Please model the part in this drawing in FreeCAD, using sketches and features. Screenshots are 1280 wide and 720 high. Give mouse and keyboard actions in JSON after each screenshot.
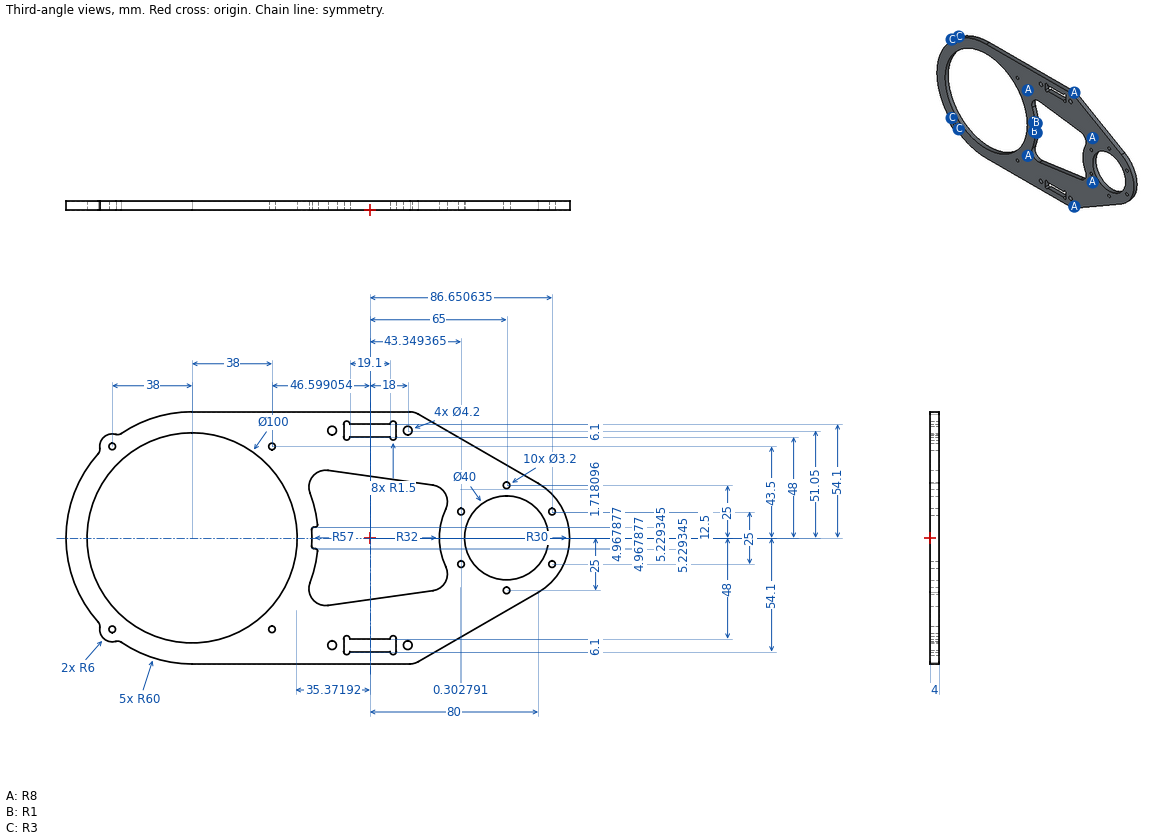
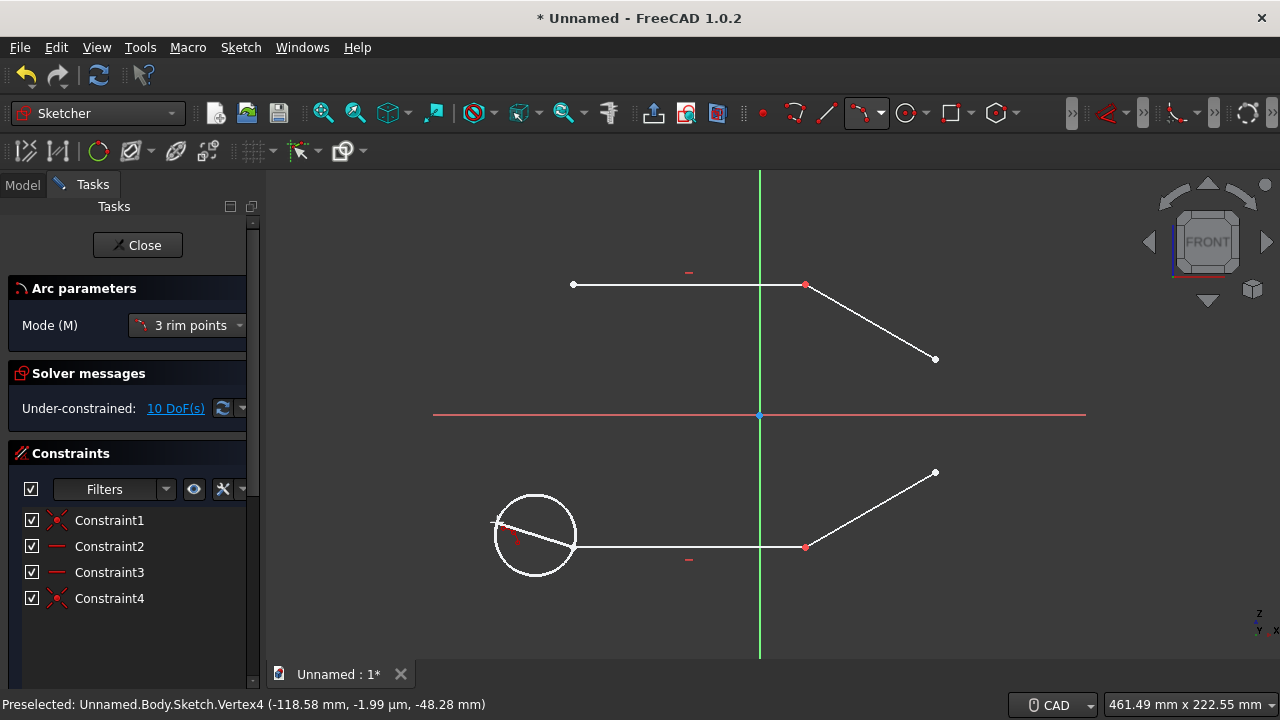
{"action": "scroll", "coordinate": [533, 541], "scroll_direction": "up", "scroll_amount": 5}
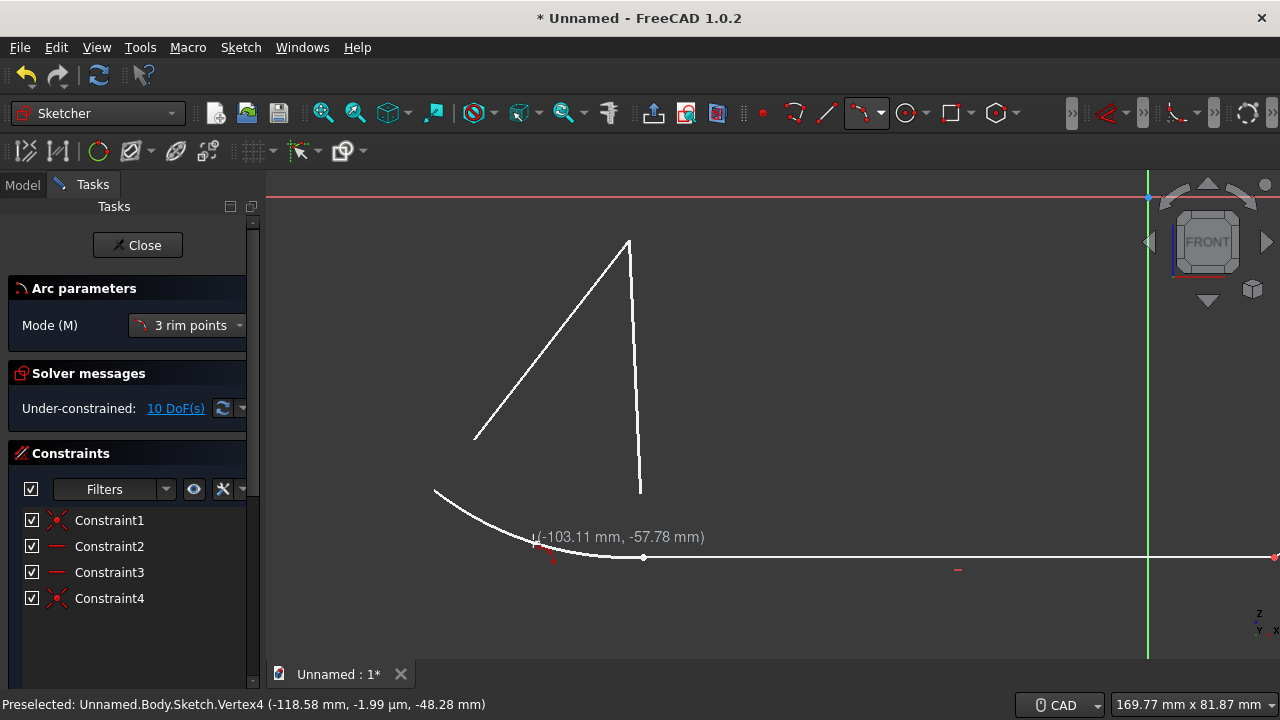
{"action": "left_click", "coordinate": [533, 538]}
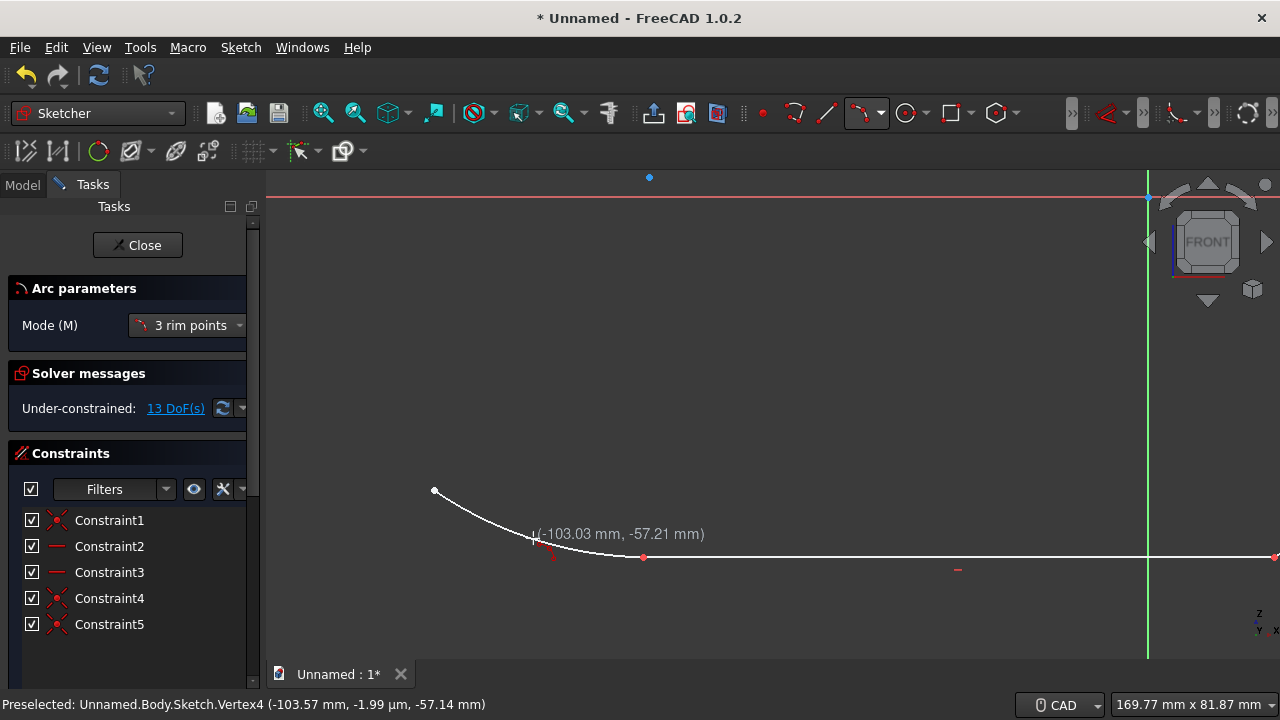
{"action": "left_click", "coordinate": [435, 491]}
{"action": "left_click", "coordinate": [383, 444]}
{"action": "left_click", "coordinate": [393, 484]}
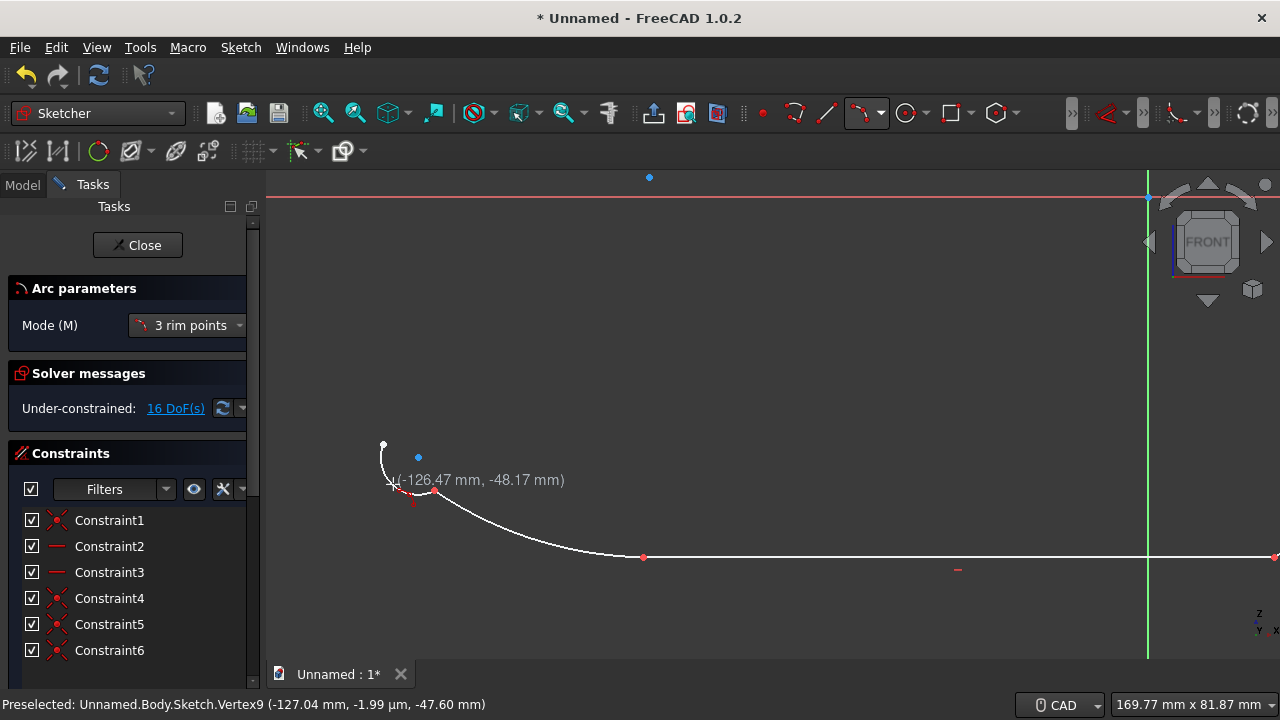
{"action": "left_click", "coordinate": [383, 445]}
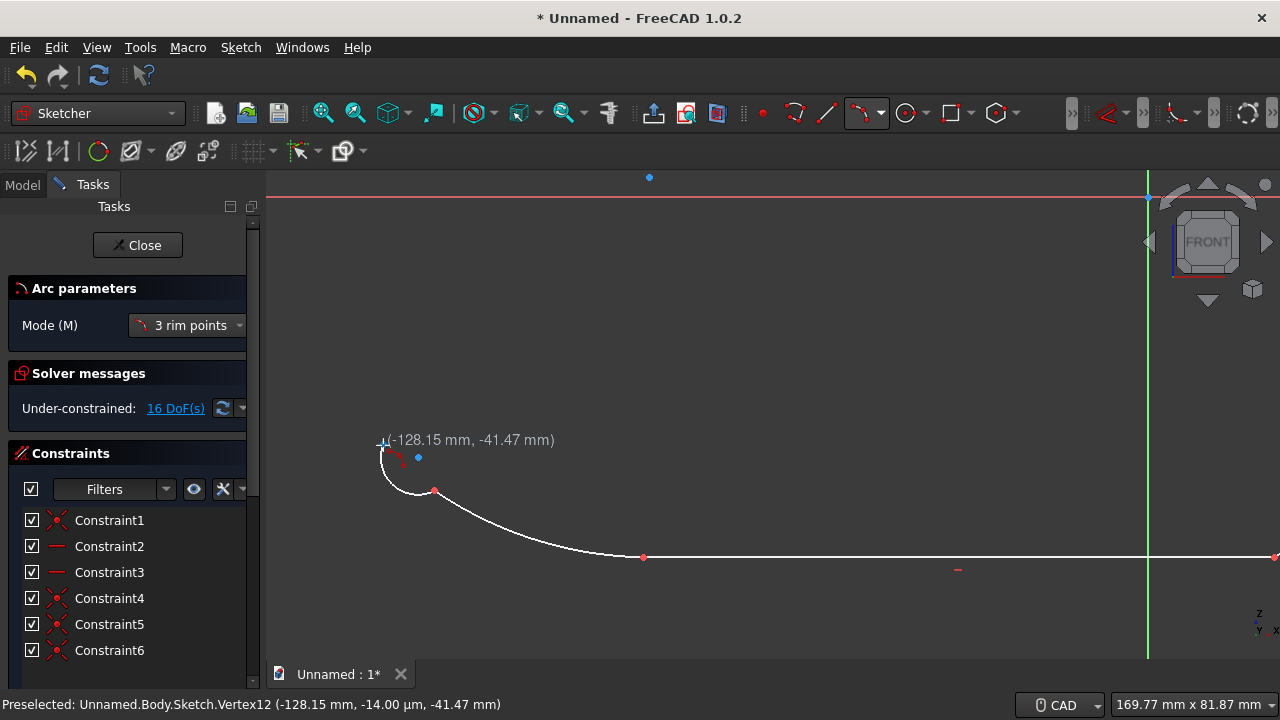
{"action": "scroll", "coordinate": [532, 541], "scroll_direction": "down", "scroll_amount": 5}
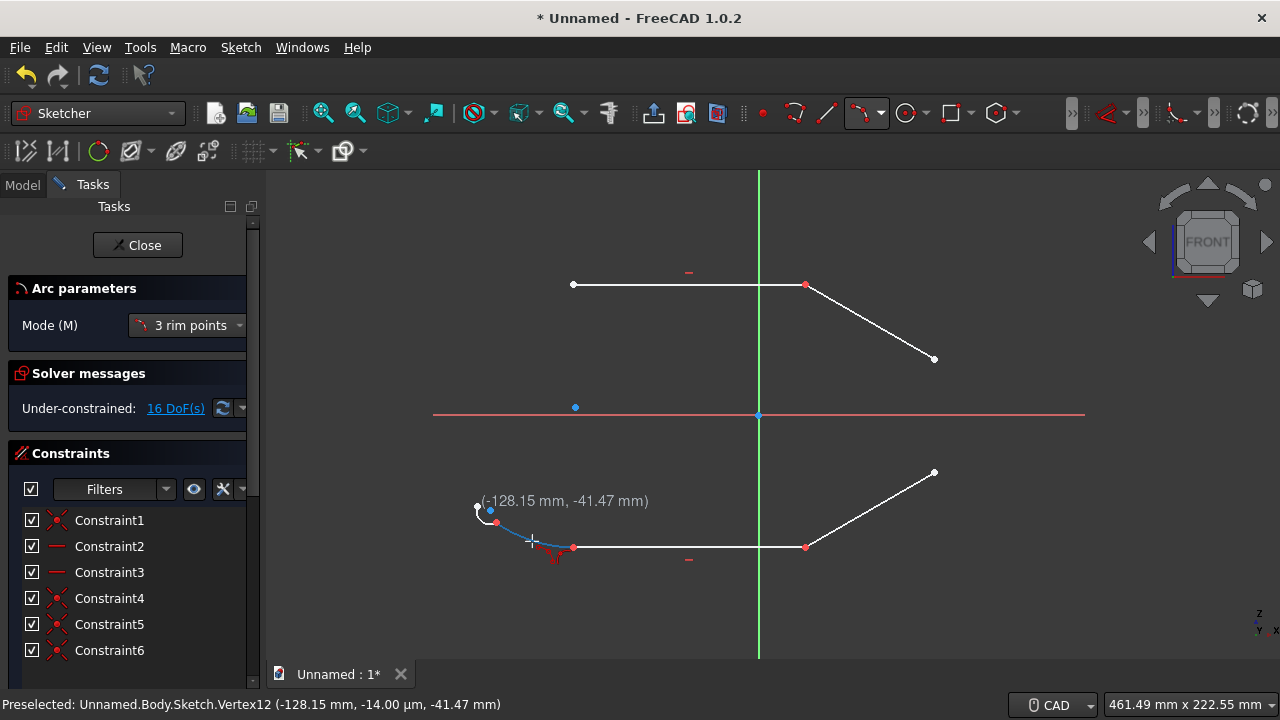
{"action": "left_click", "coordinate": [477, 324]}
{"action": "left_click", "coordinate": [443, 395]}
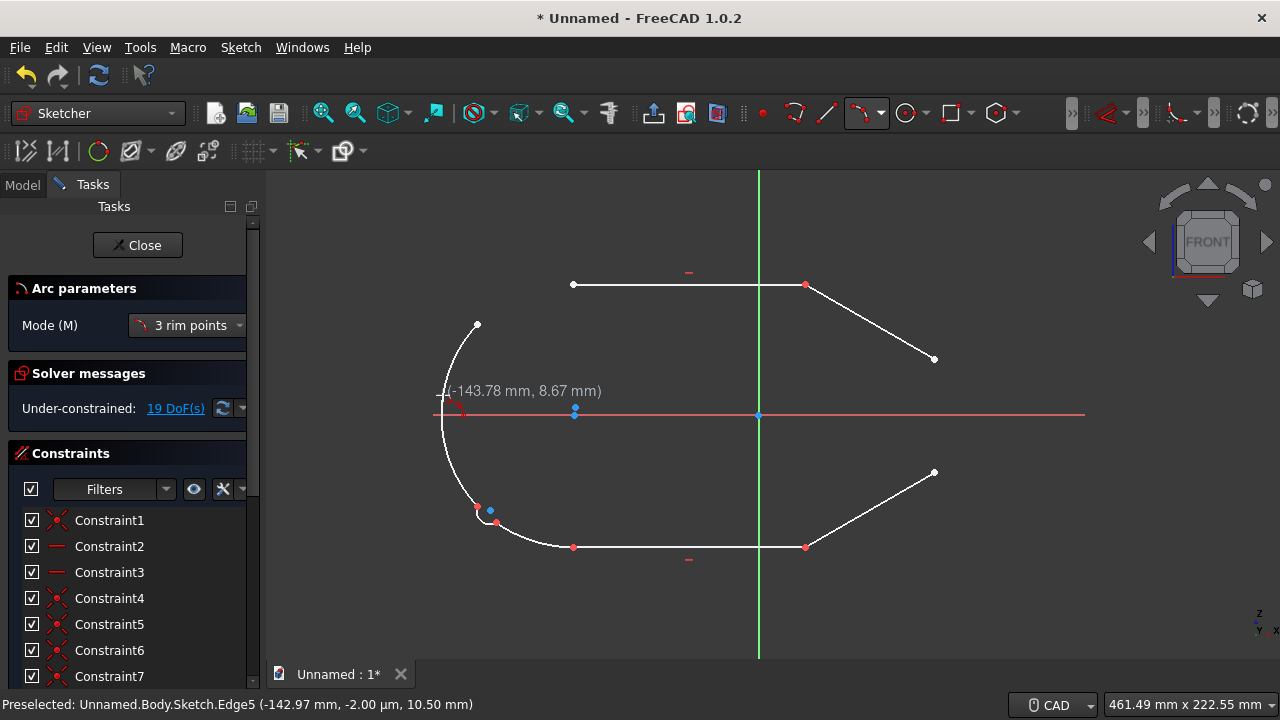
{"action": "left_click", "coordinate": [477, 325]}
{"action": "left_click", "coordinate": [496, 308]}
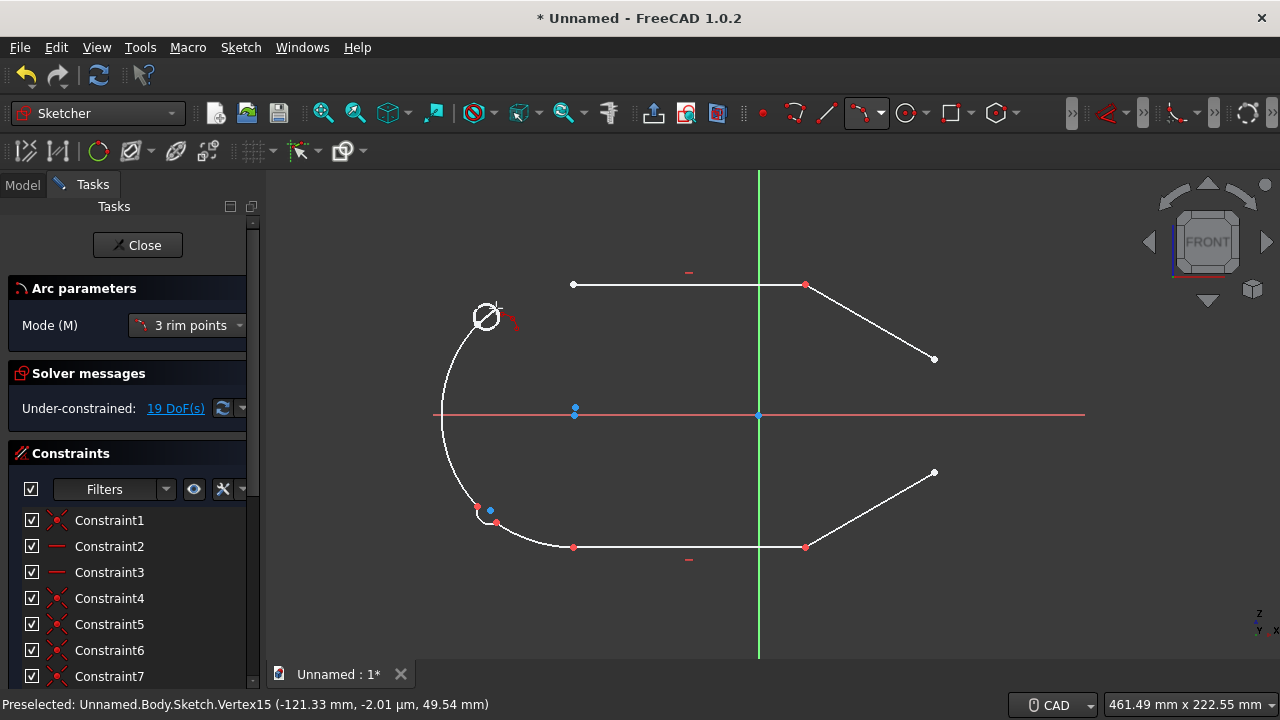
{"action": "scroll", "coordinate": [481, 310], "scroll_direction": "up", "scroll_amount": 3}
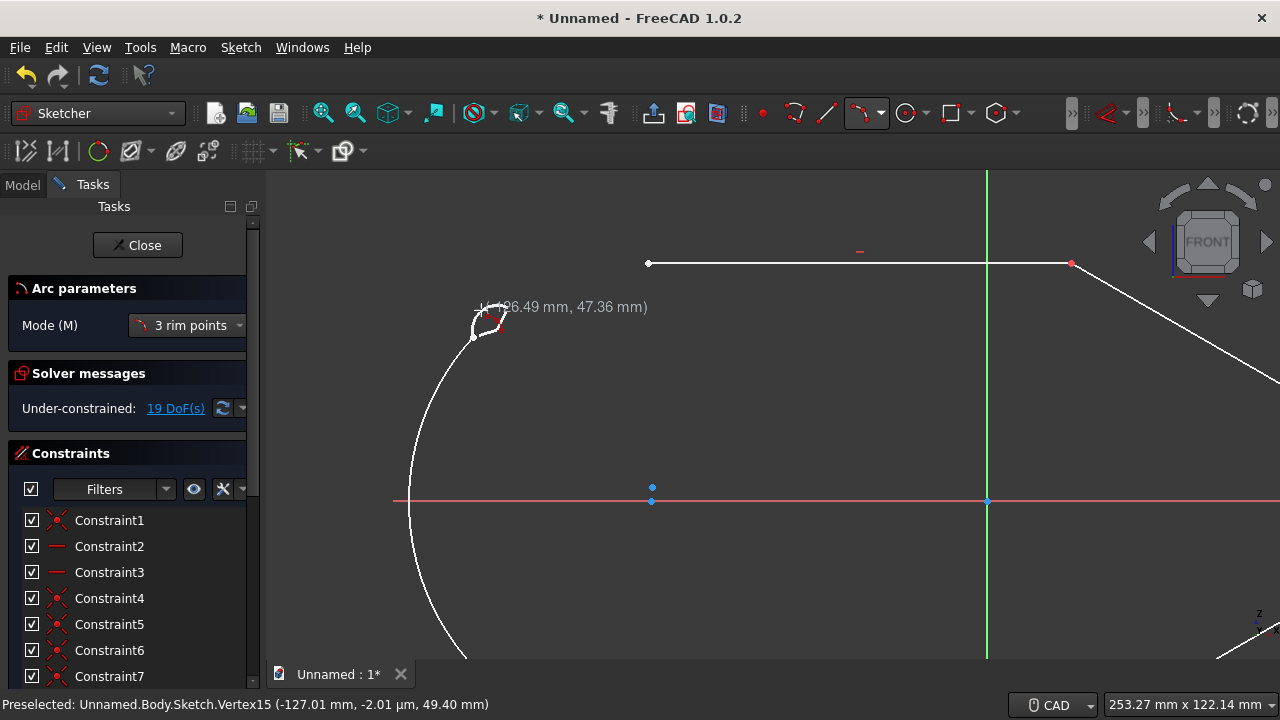
{"action": "left_click", "coordinate": [481, 309]}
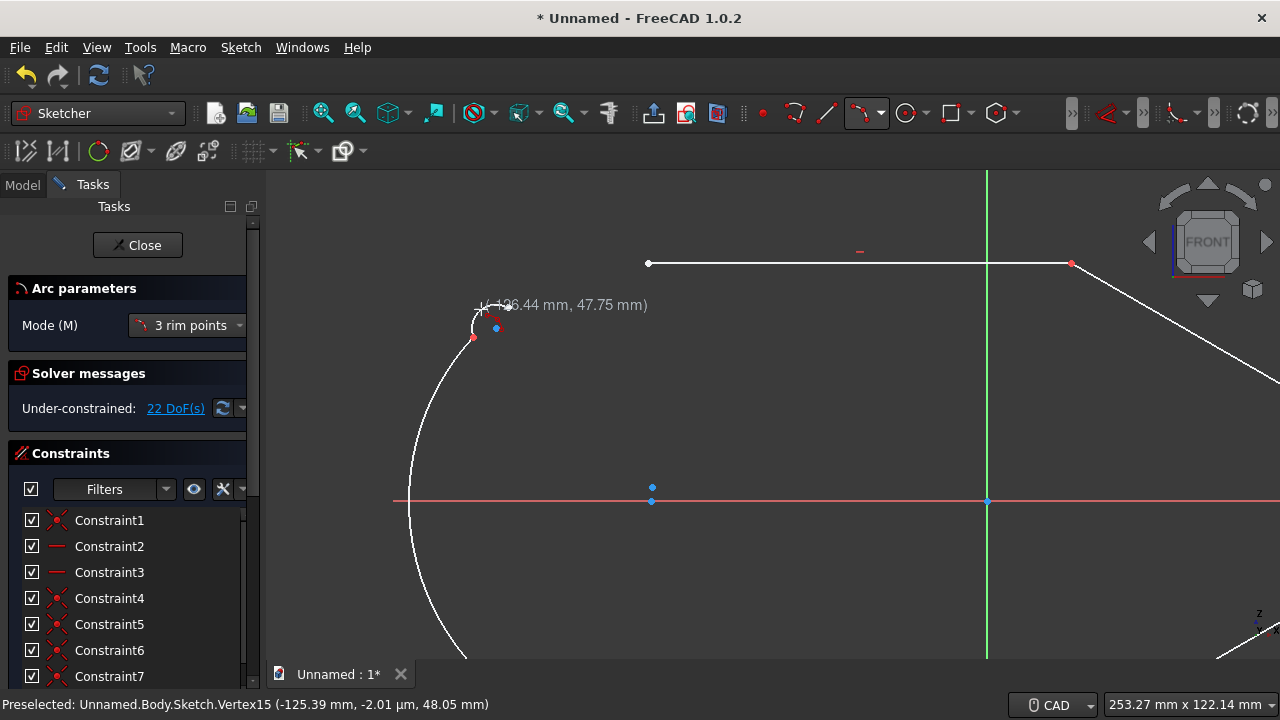
{"action": "left_click", "coordinate": [508, 308]}
{"action": "left_click", "coordinate": [649, 263]}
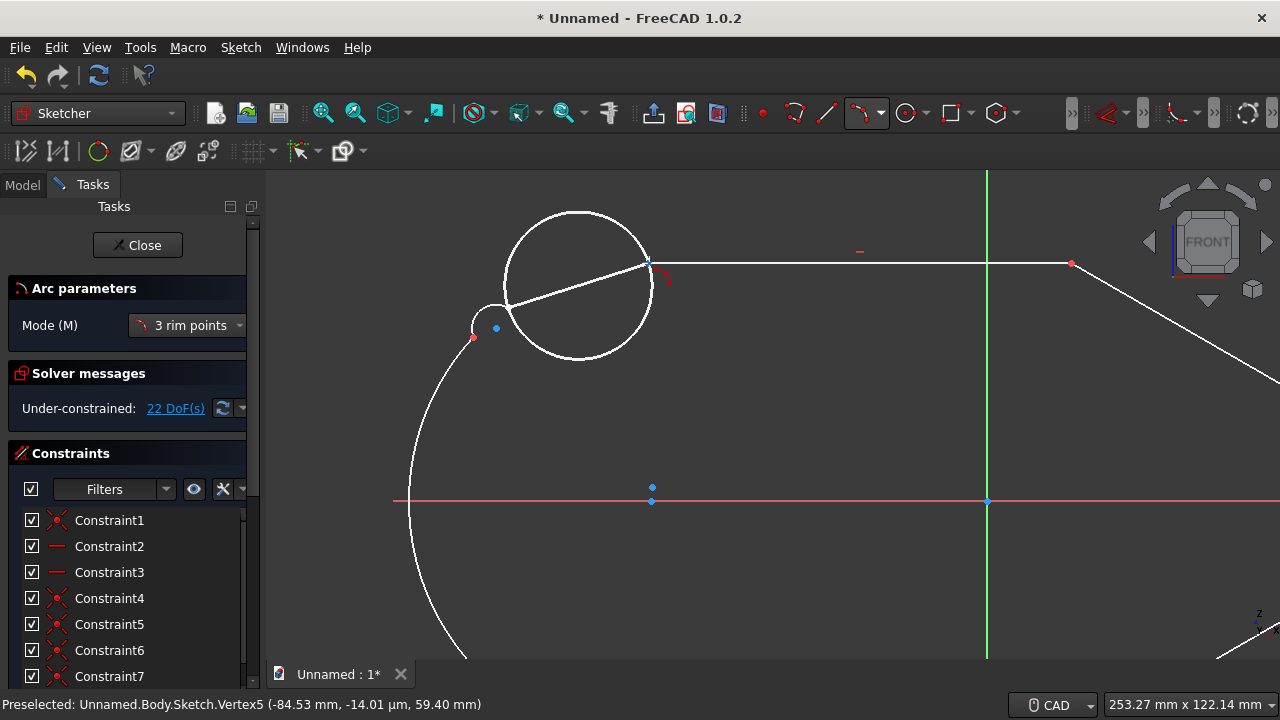
{"action": "scroll", "coordinate": [575, 273], "scroll_direction": "up", "scroll_amount": 2}